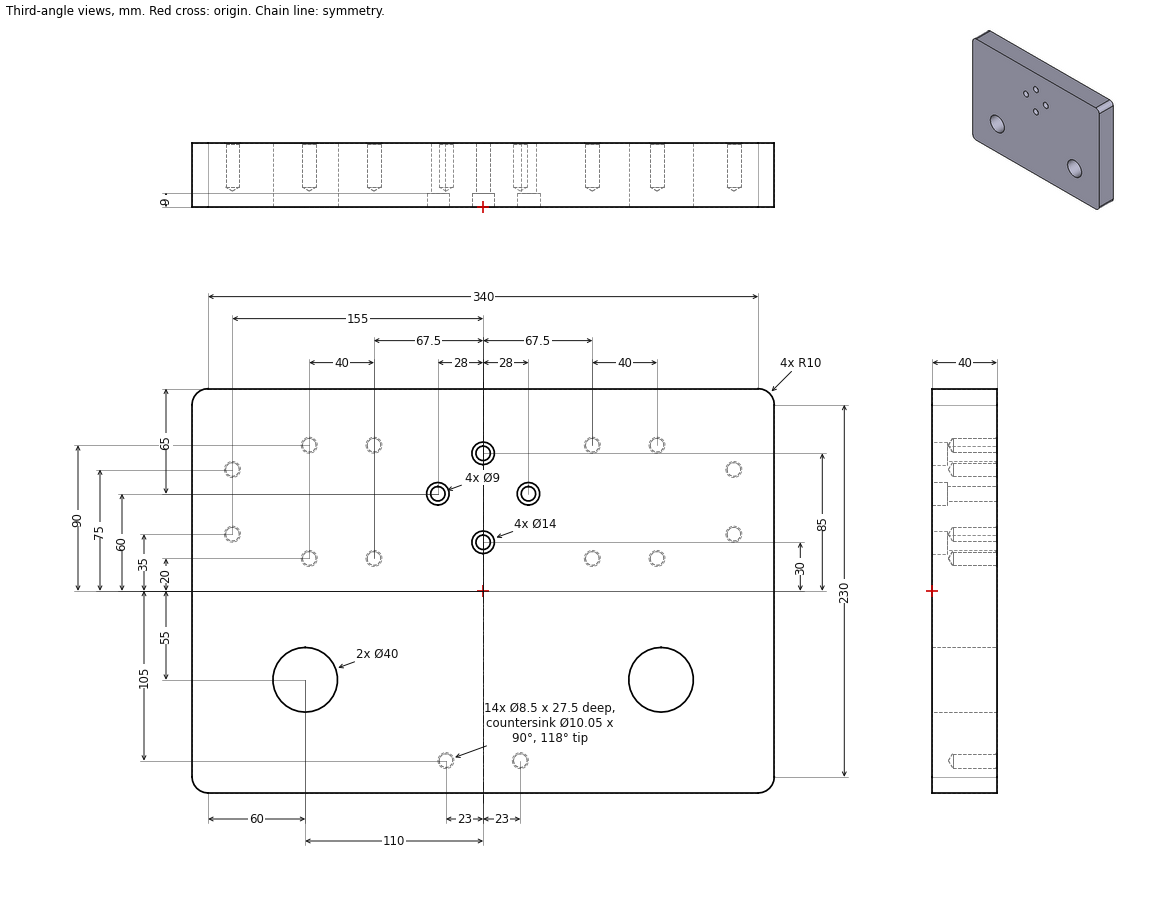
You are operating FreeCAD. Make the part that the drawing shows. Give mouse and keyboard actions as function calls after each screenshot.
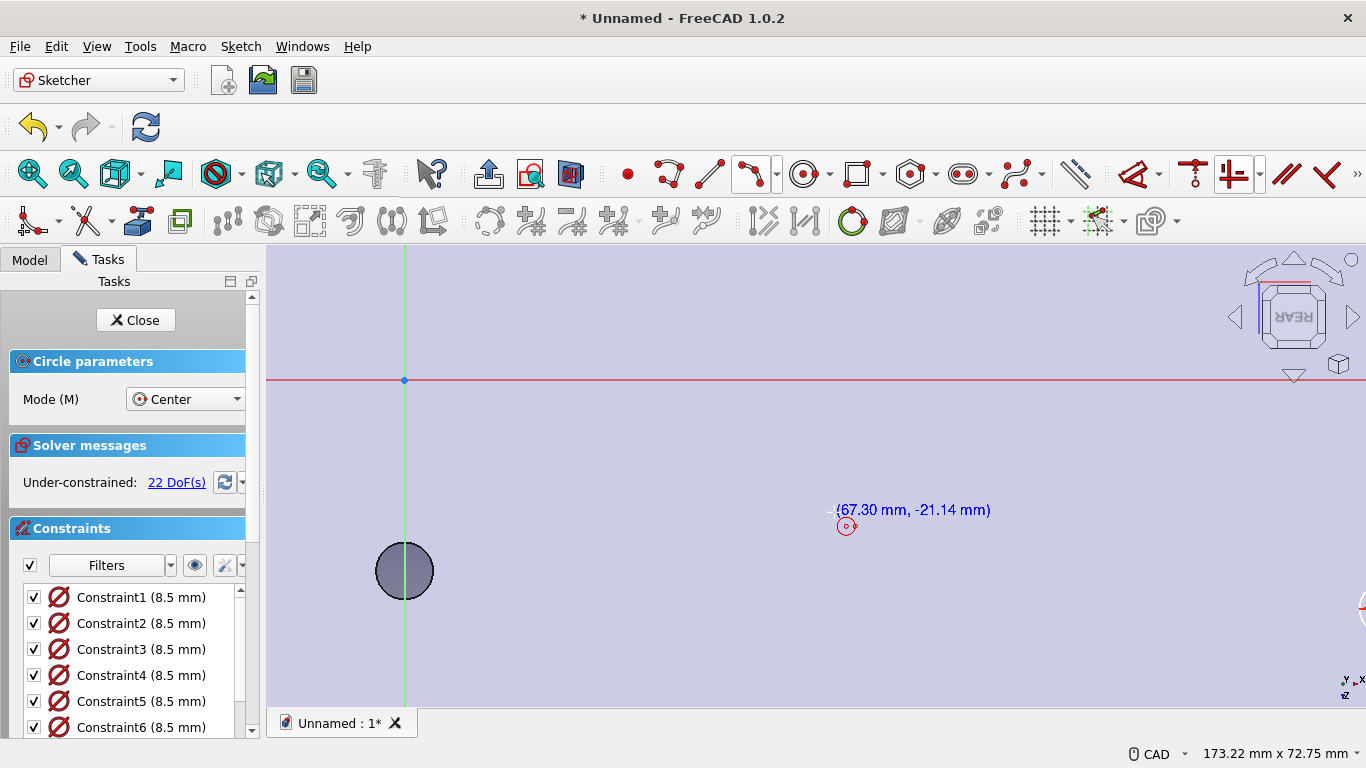
scroll(834, 512, down, 8)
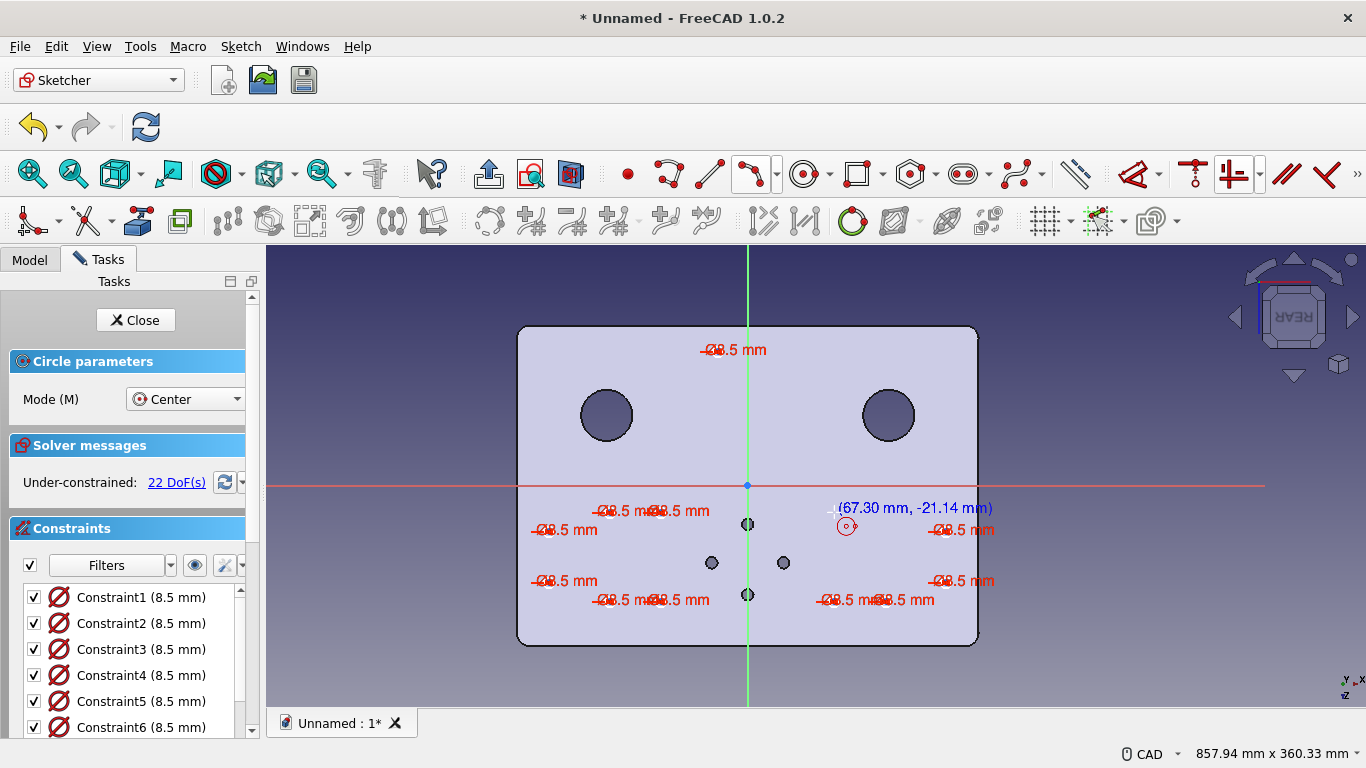
click(834, 512)
move(838, 508)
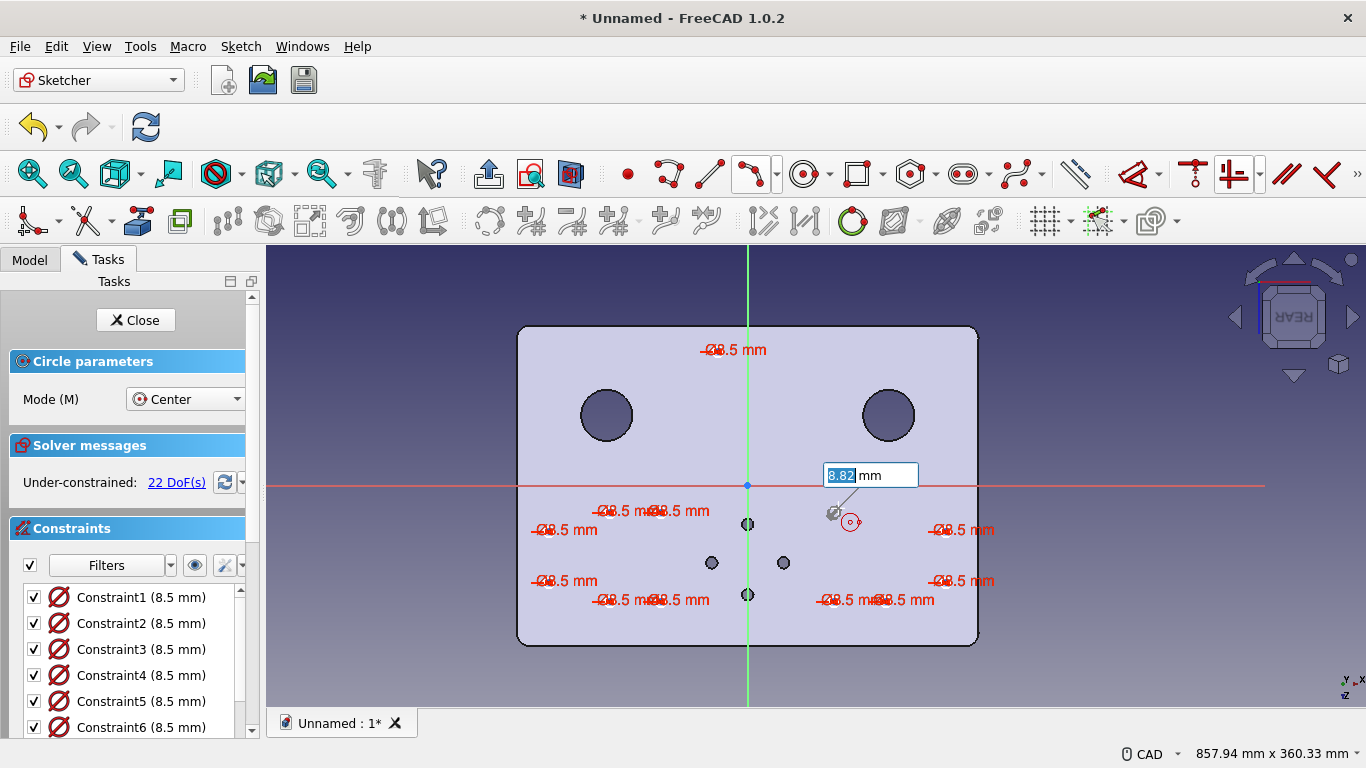
text(8.5)
key(Return)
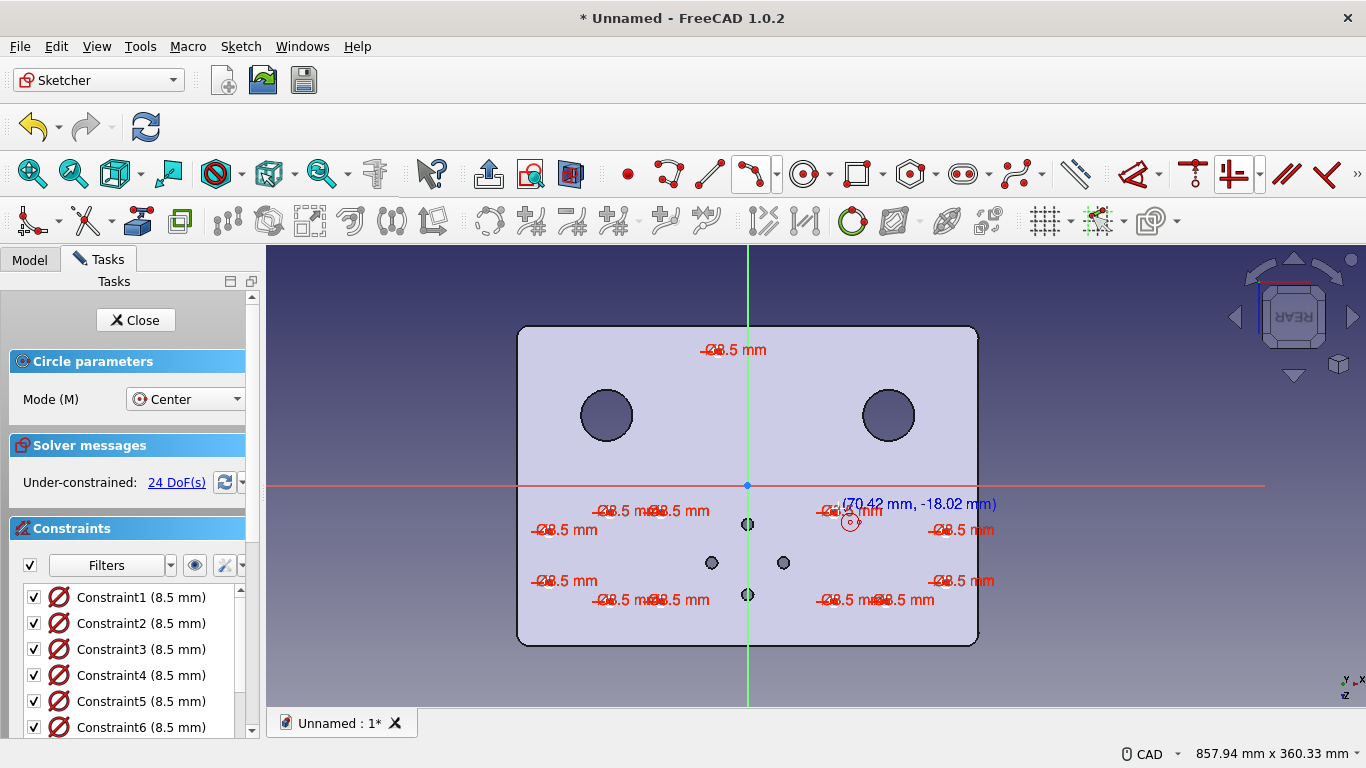
scroll(886, 512, up, 8)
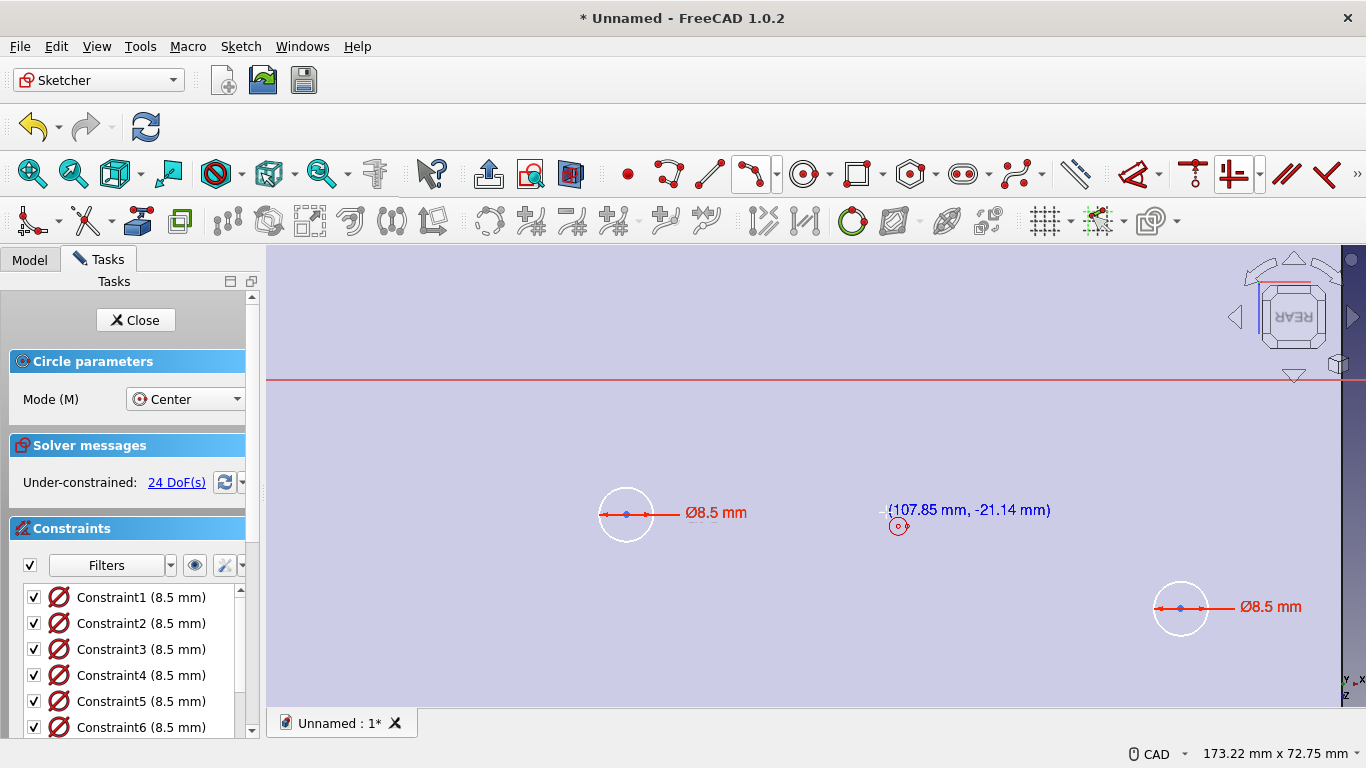
scroll(886, 512, down, 8)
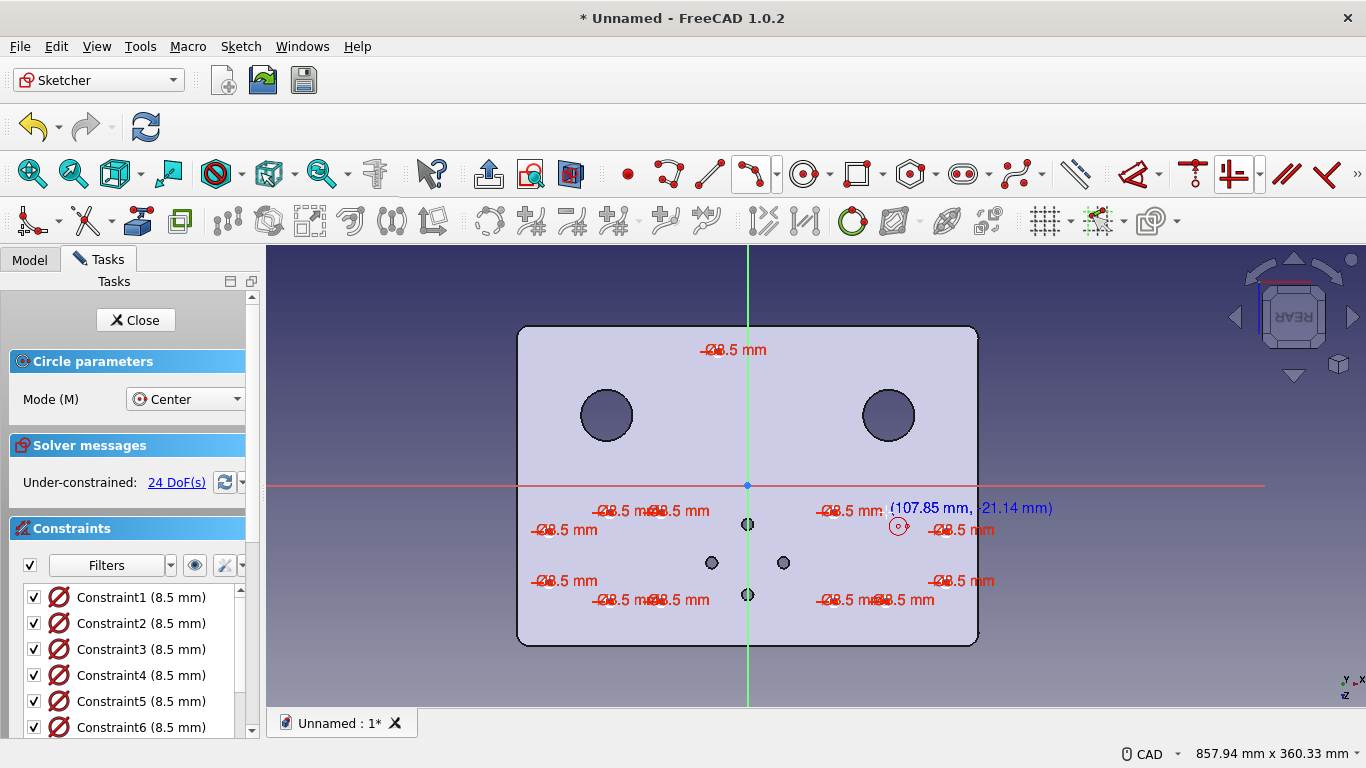
click(886, 512)
move(889, 508)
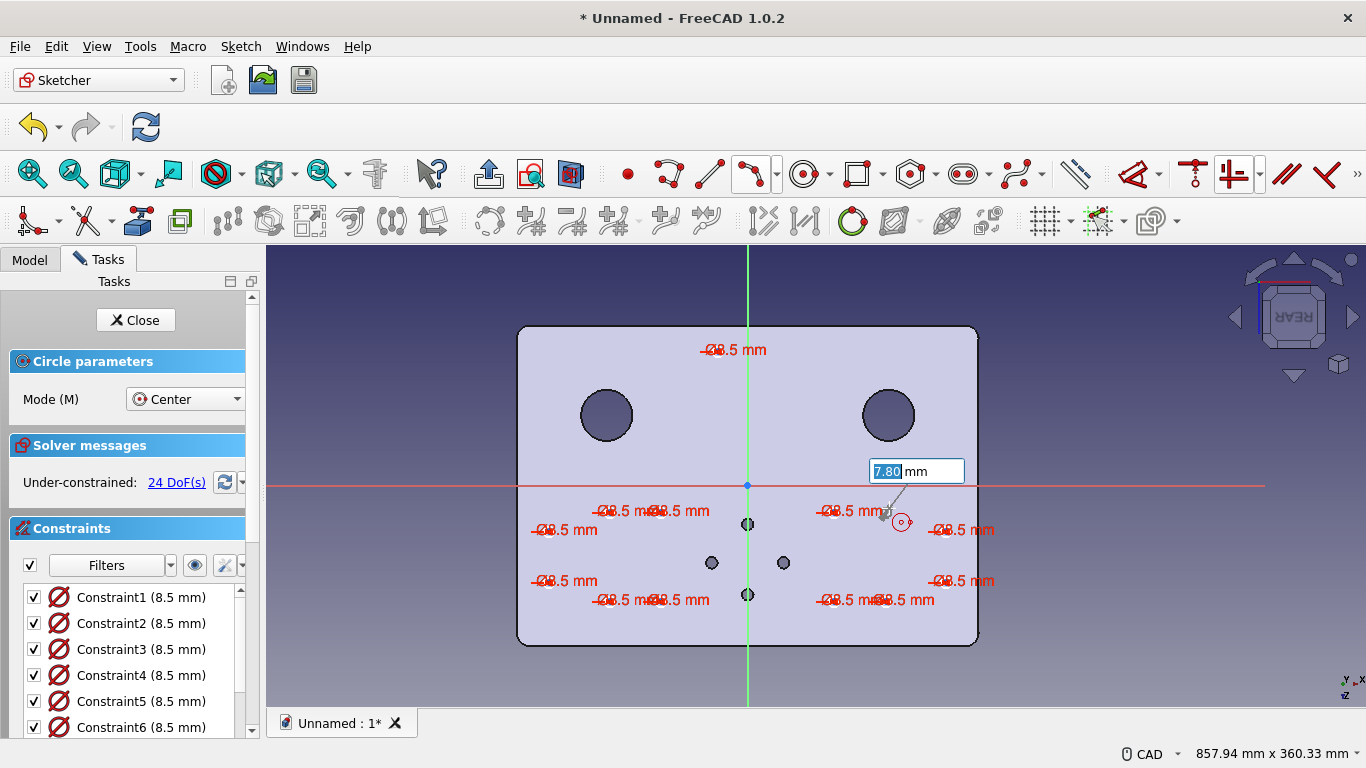
text(8.5)
key(Return)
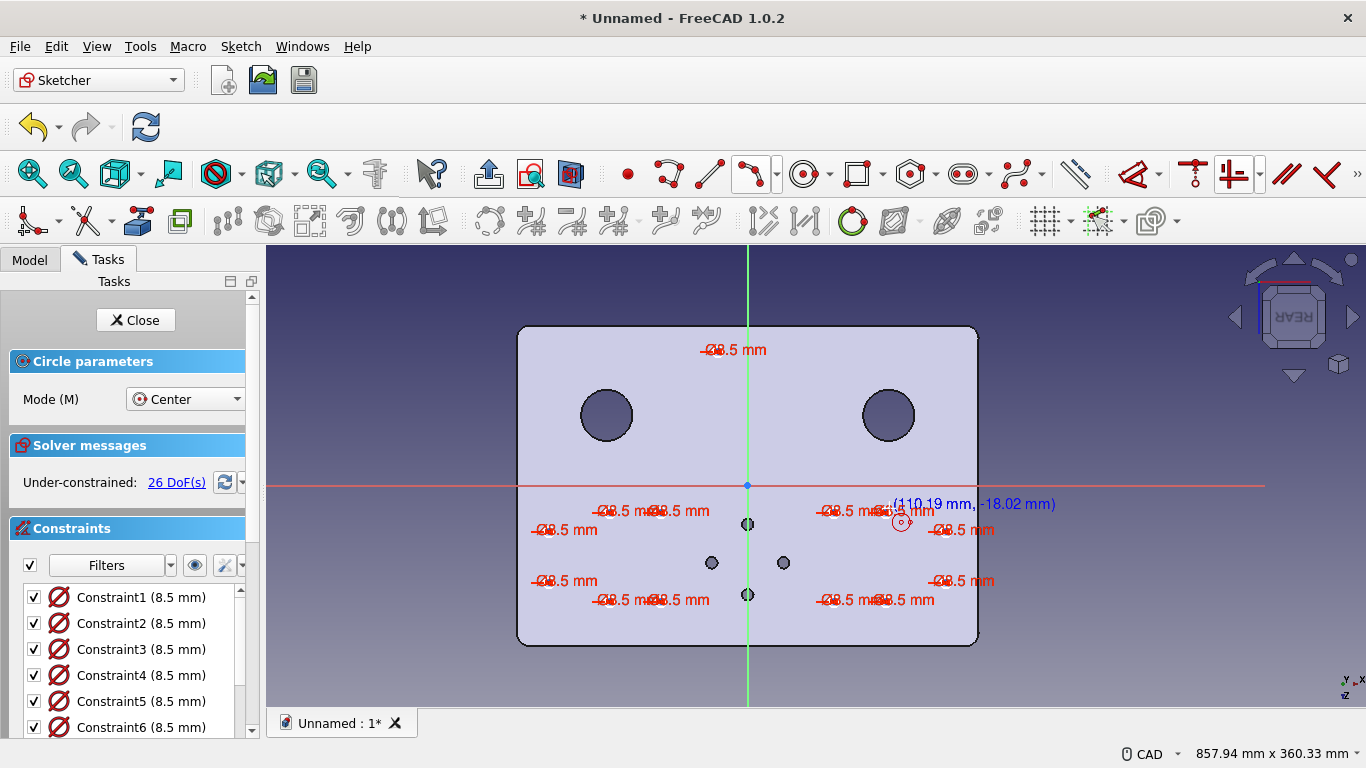
scroll(777, 351, up, 8)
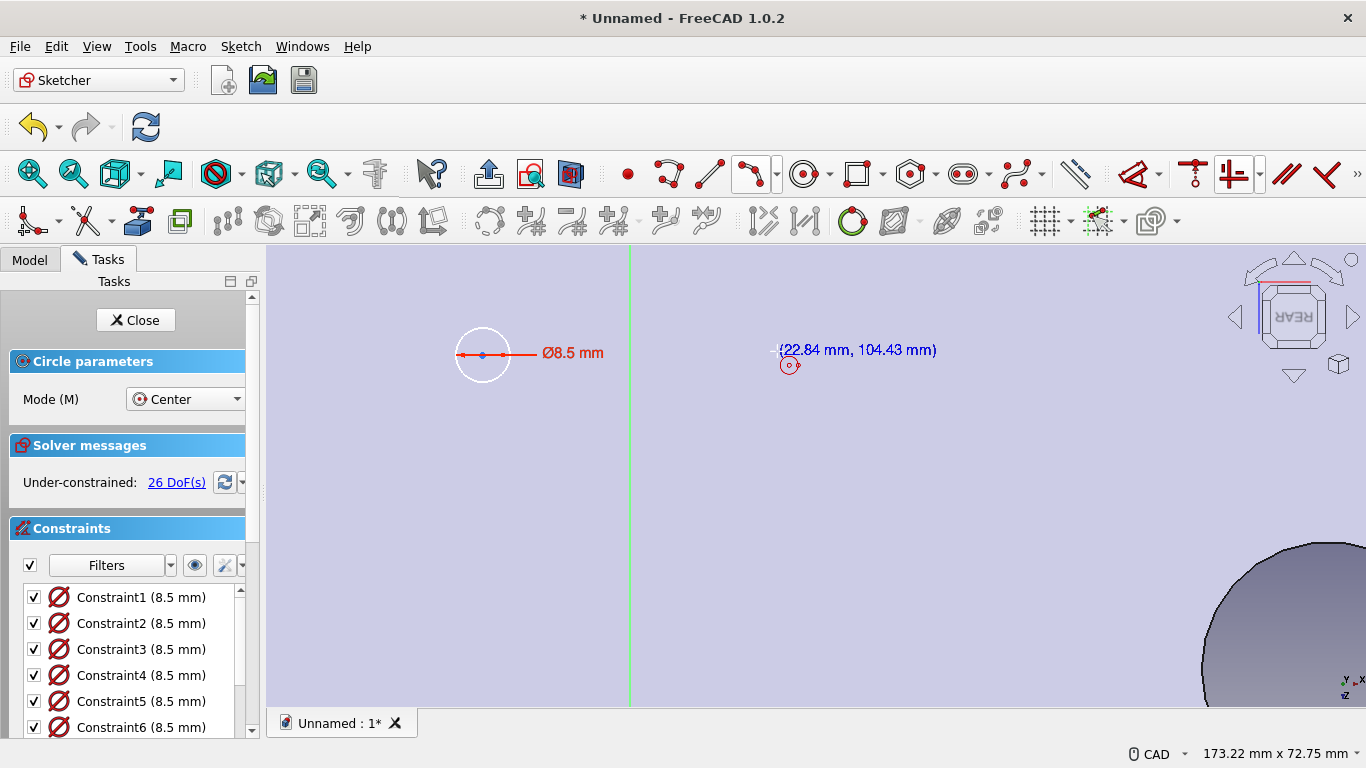
scroll(777, 351, down, 8)